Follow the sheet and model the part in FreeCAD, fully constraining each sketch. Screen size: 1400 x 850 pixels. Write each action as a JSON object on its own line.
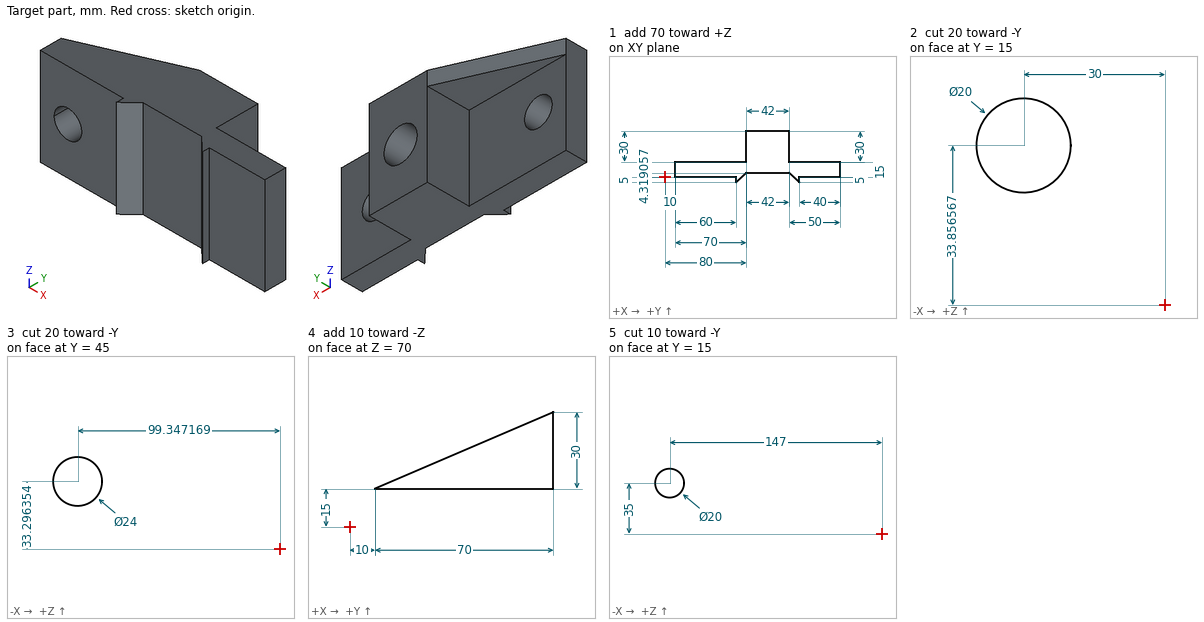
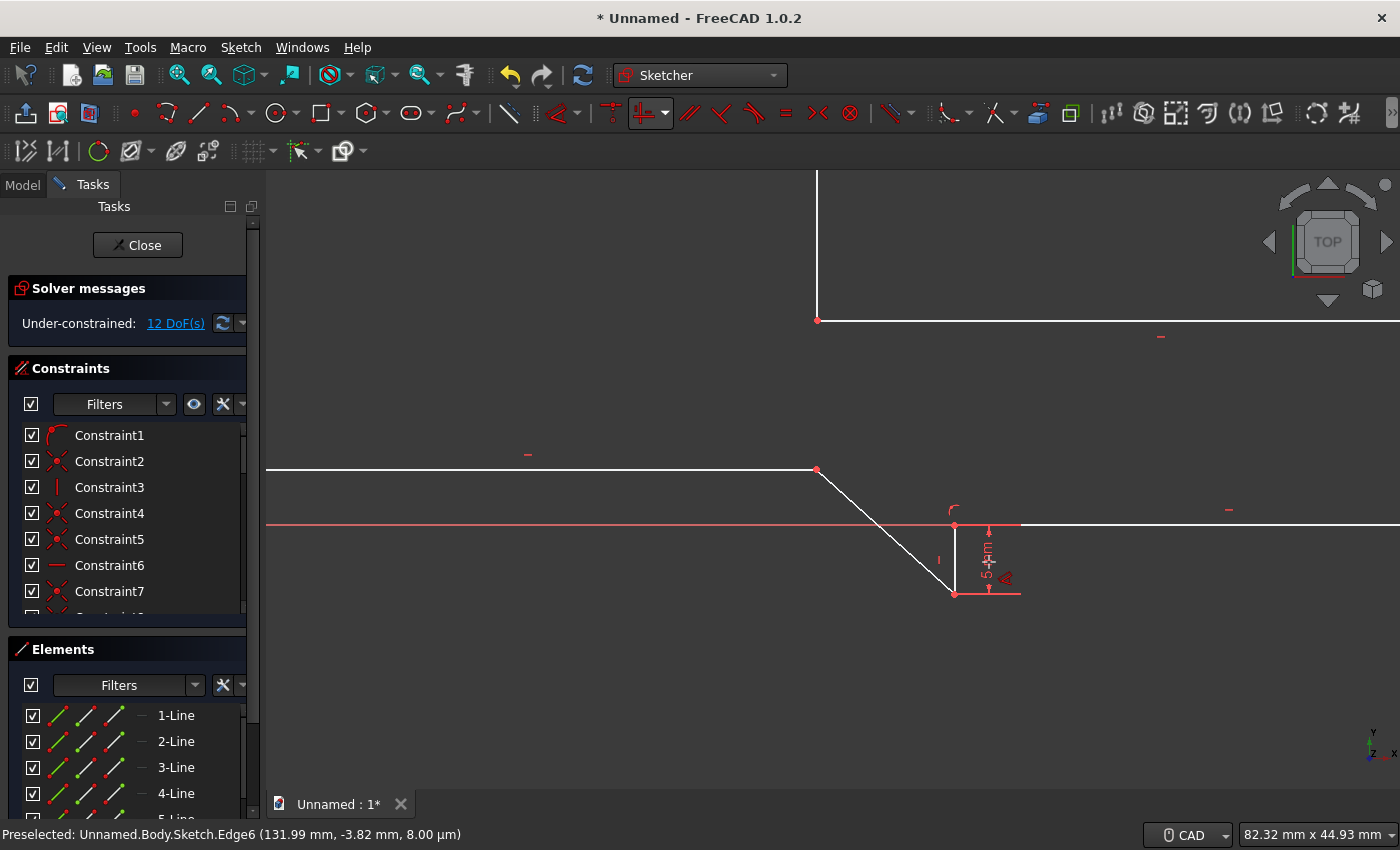
{"action": "scroll", "coordinate": [956, 578], "scroll_direction": "down", "scroll_amount": 6}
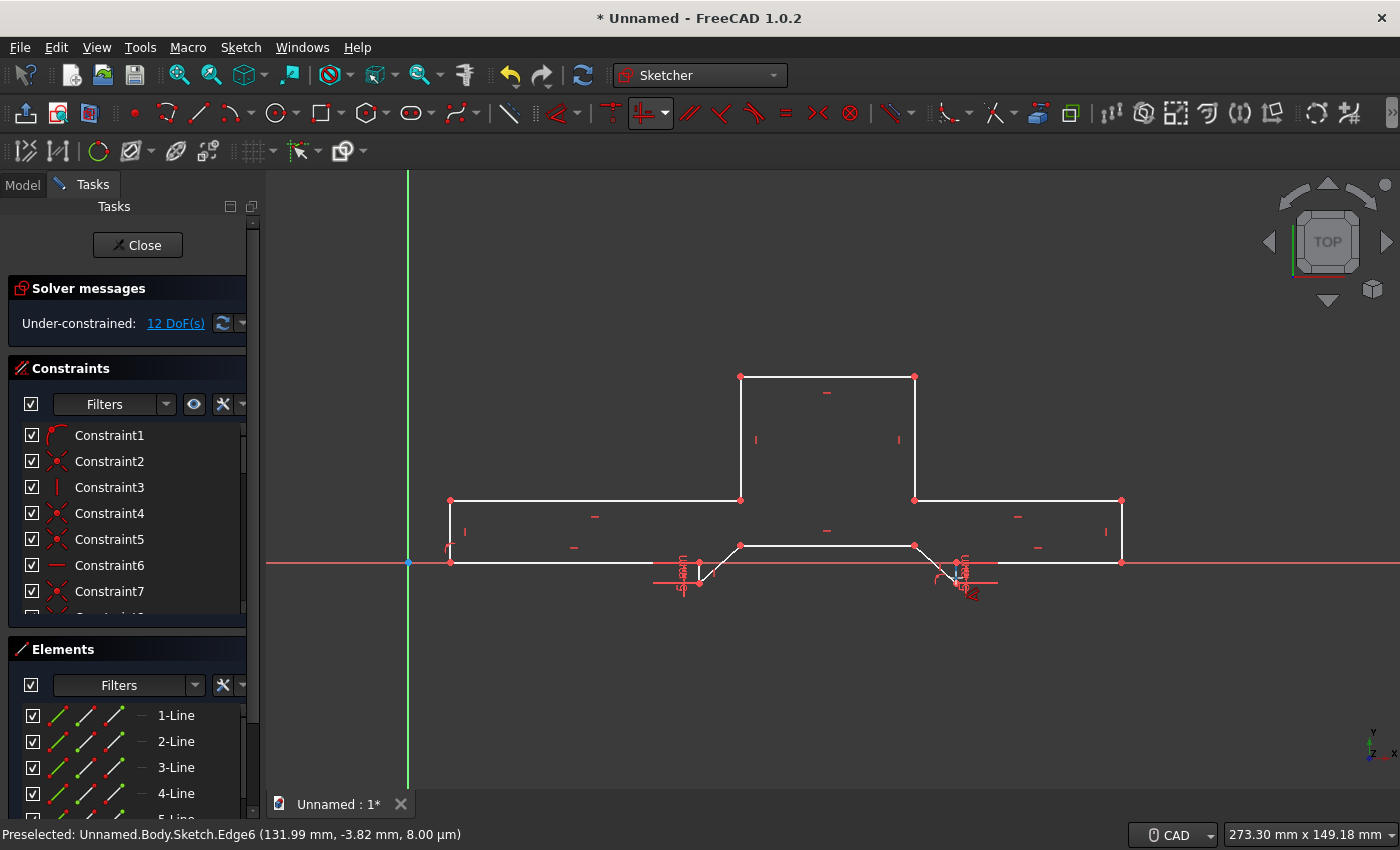
{"action": "left_click", "coordinate": [525, 563]}
{"action": "left_click", "coordinate": [575, 597]}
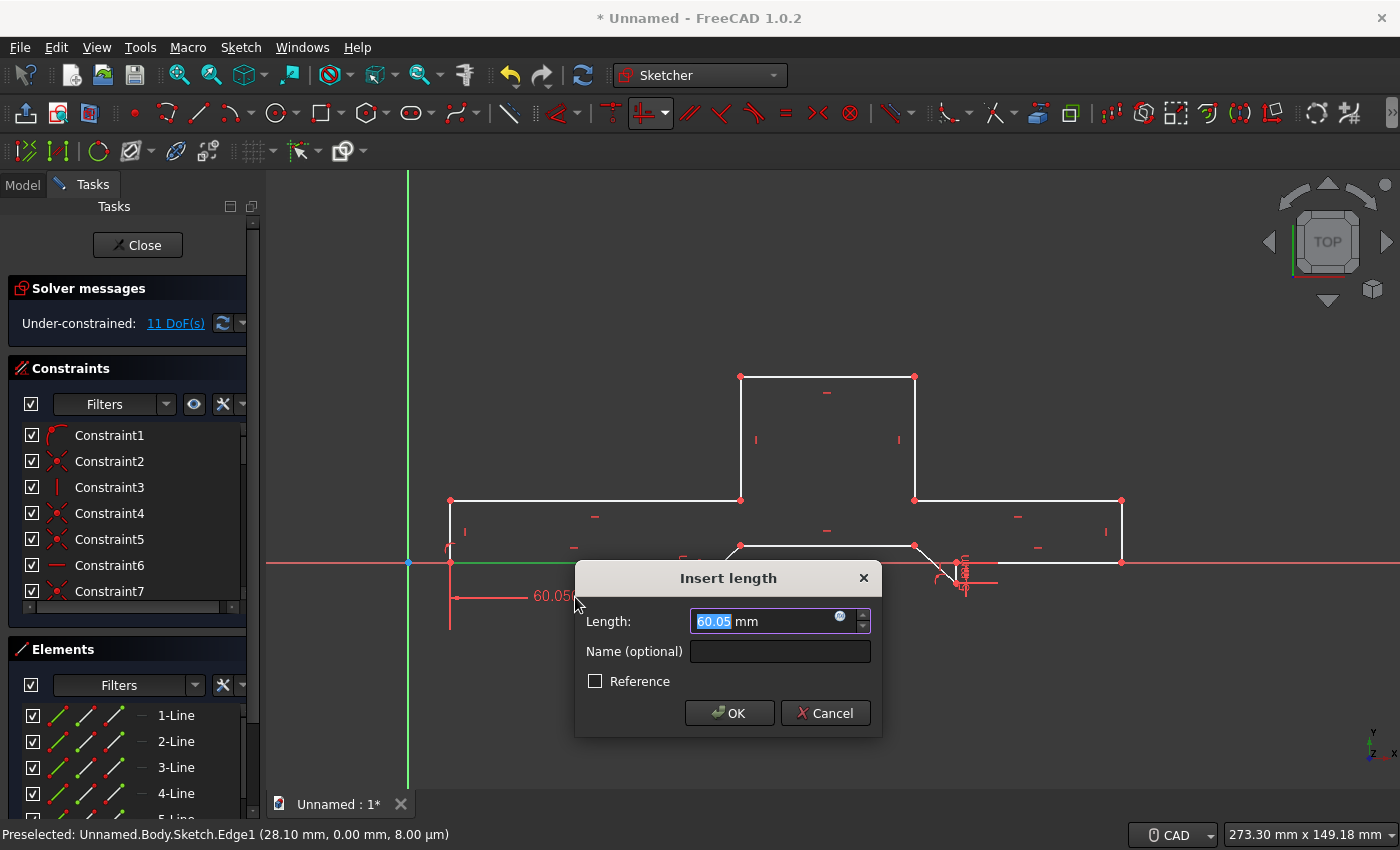
{"action": "type", "text": "60"}
{"action": "key", "text": "Return"}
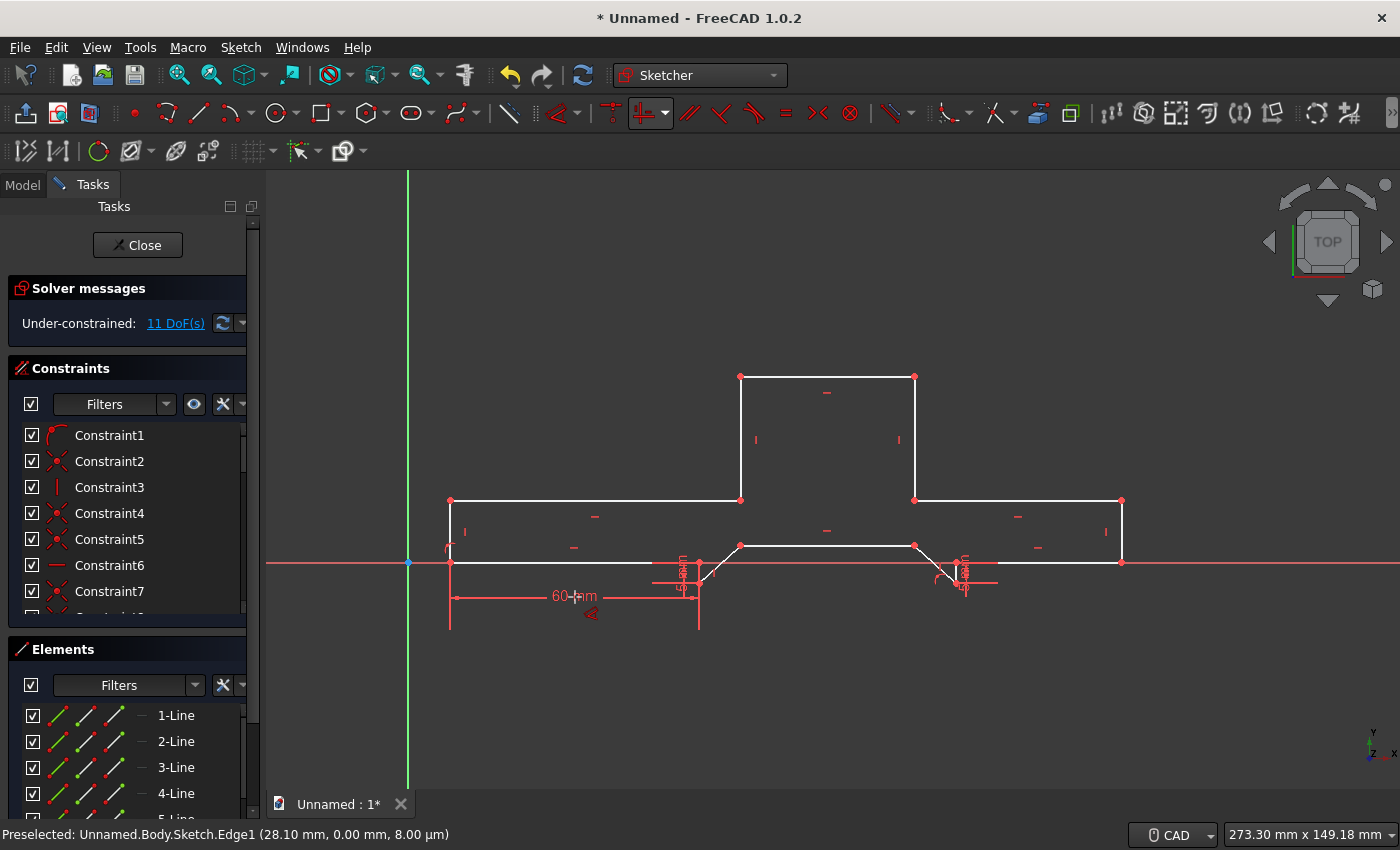
{"action": "left_click", "coordinate": [793, 546]}
{"action": "left_click", "coordinate": [828, 580]}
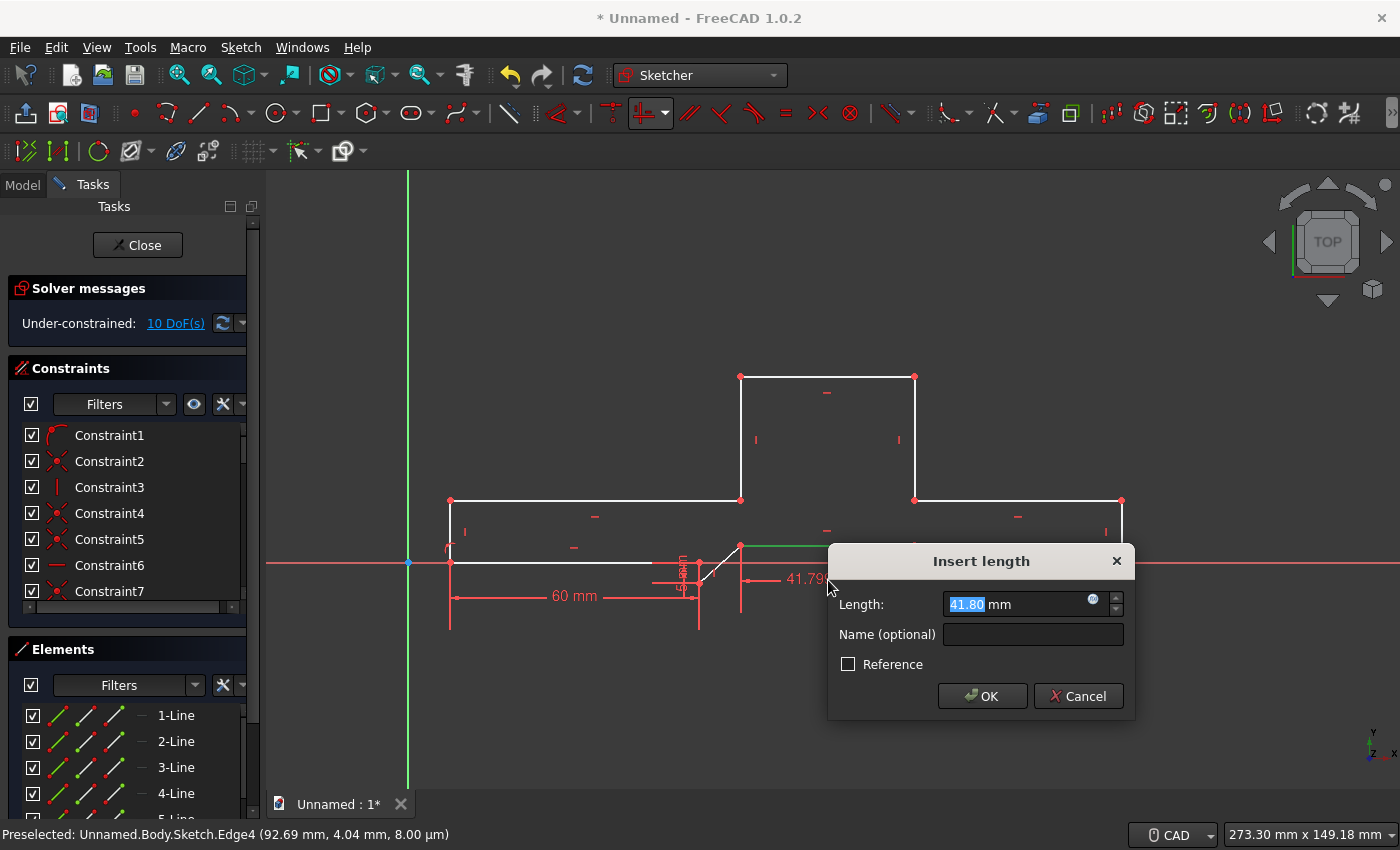
{"action": "type", "text": "42"}
{"action": "key", "text": "Return"}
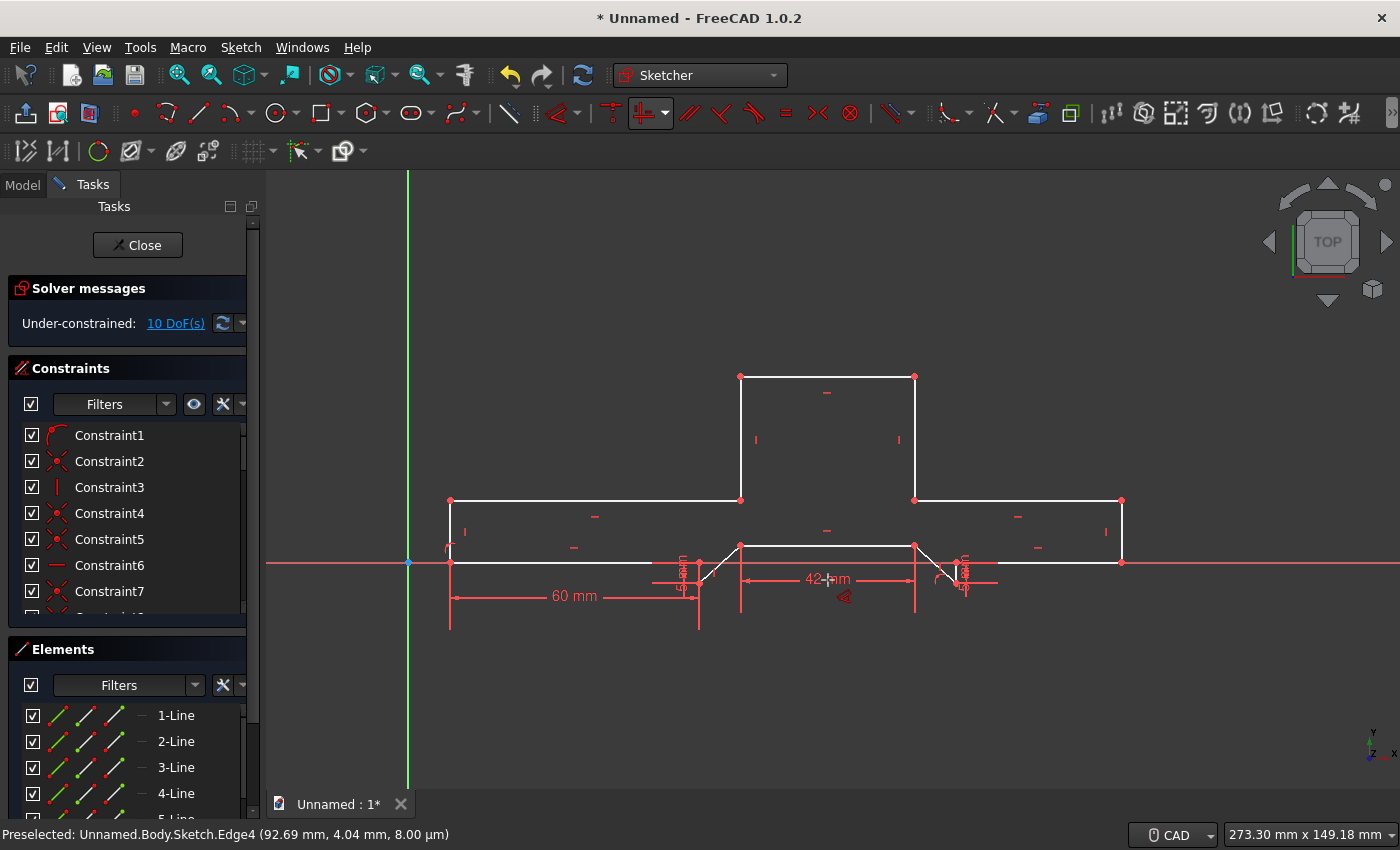
{"action": "left_click", "coordinate": [1006, 563]}
{"action": "left_click", "coordinate": [1039, 597]}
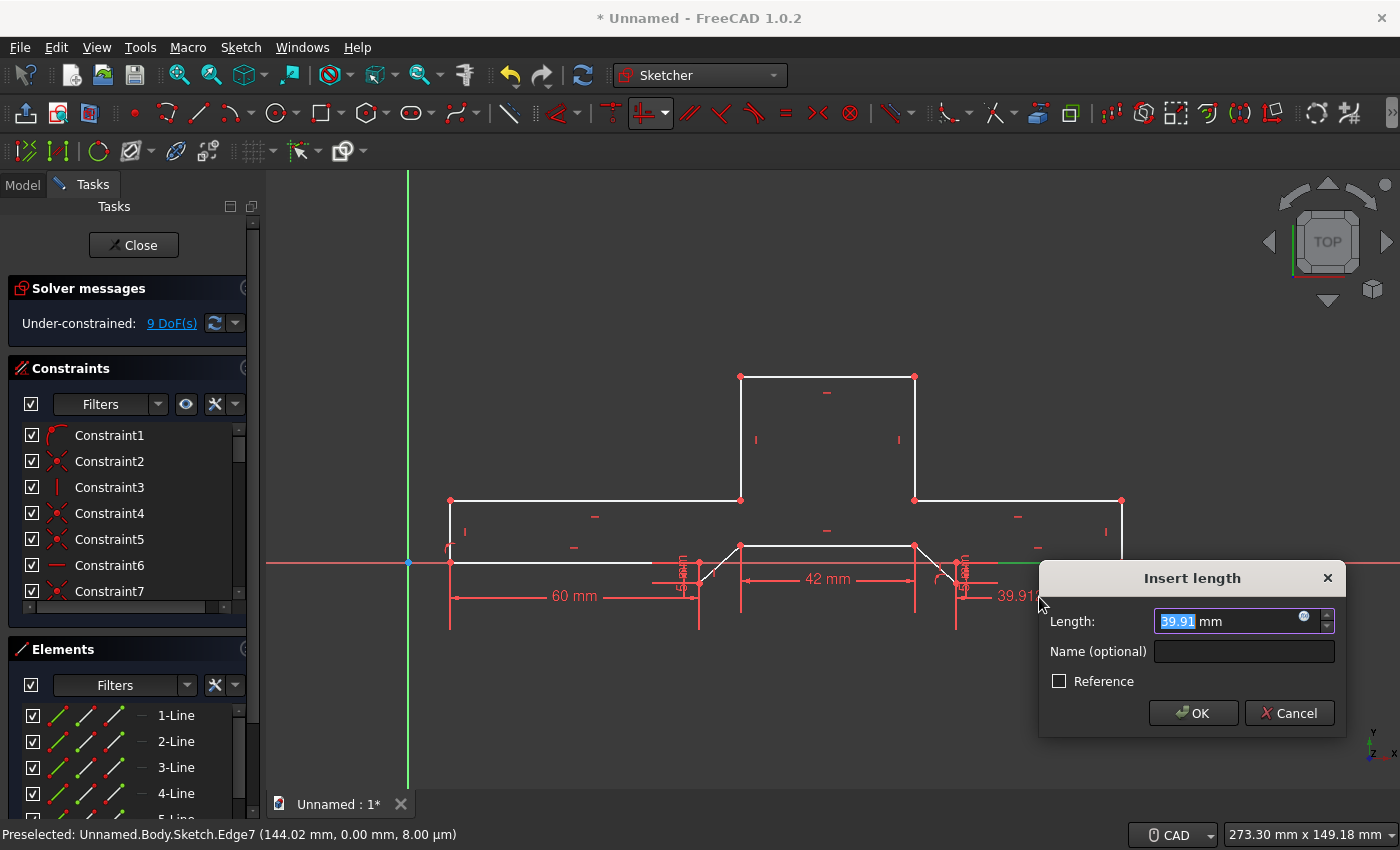
{"action": "type", "text": "40"}
{"action": "key", "text": "Return"}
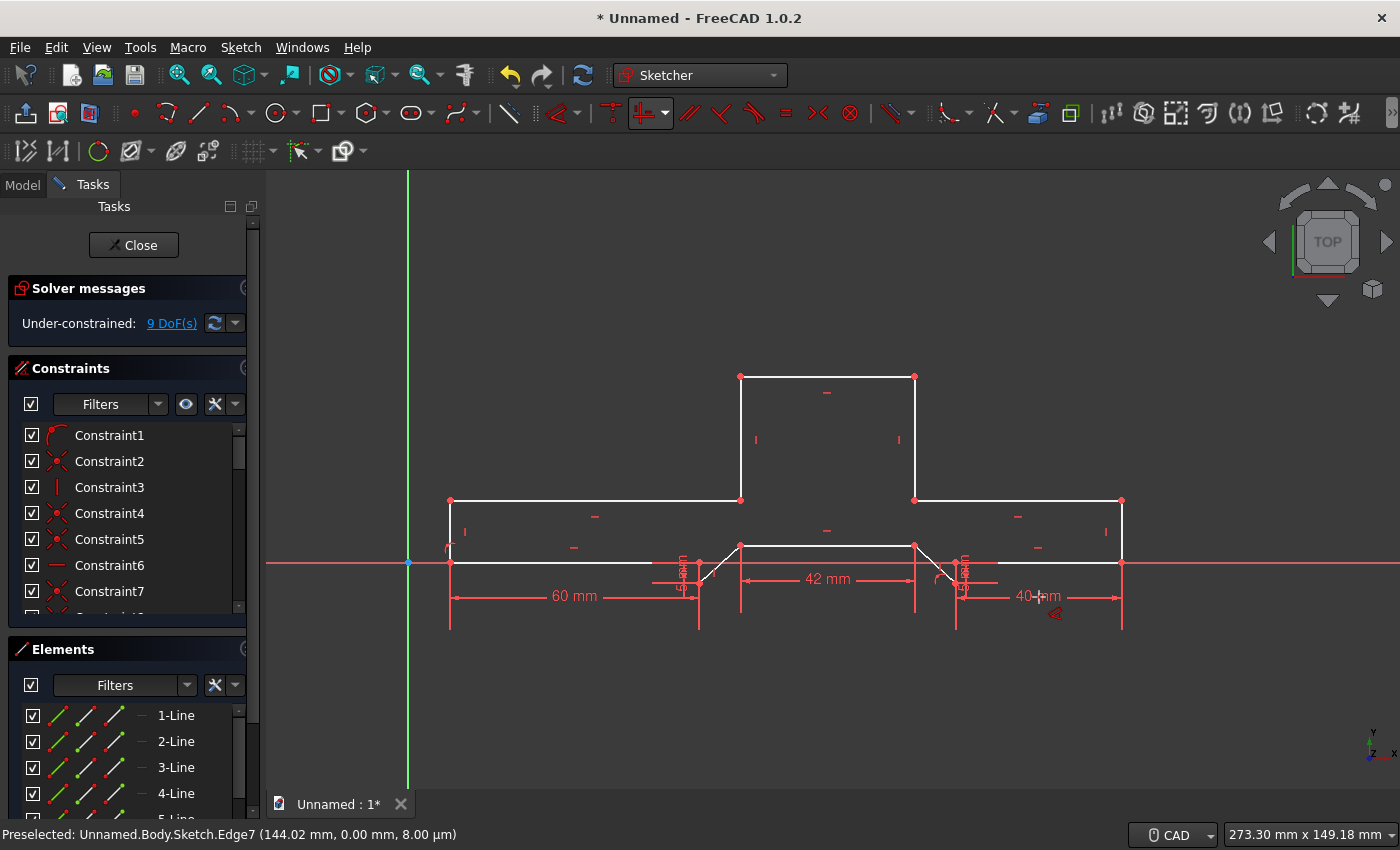
{"action": "left_click", "coordinate": [1122, 544]}
{"action": "left_click", "coordinate": [1156, 532]}